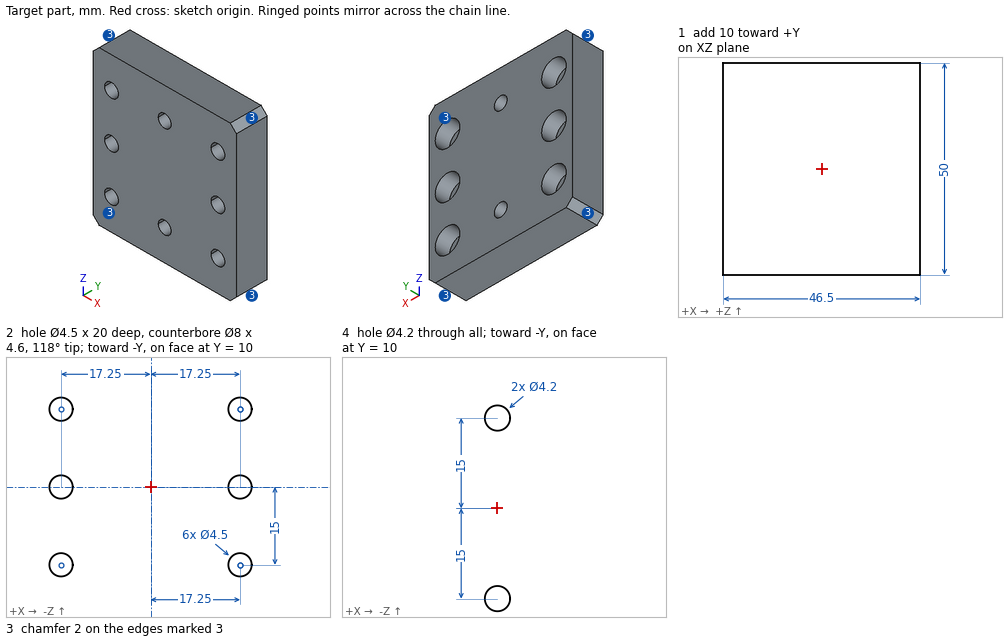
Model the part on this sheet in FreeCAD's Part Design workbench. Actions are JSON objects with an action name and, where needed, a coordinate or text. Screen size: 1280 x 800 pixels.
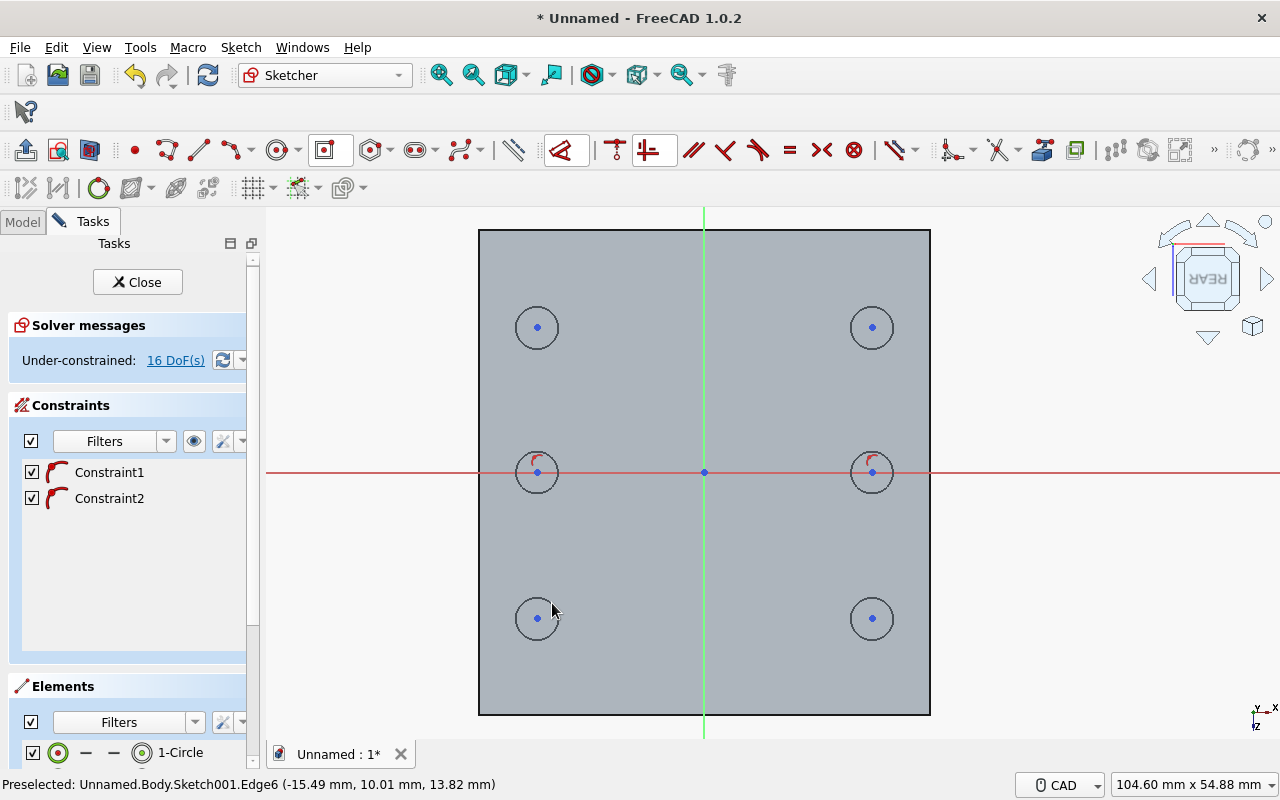
{"action": "left_click", "coordinate": [887, 604]}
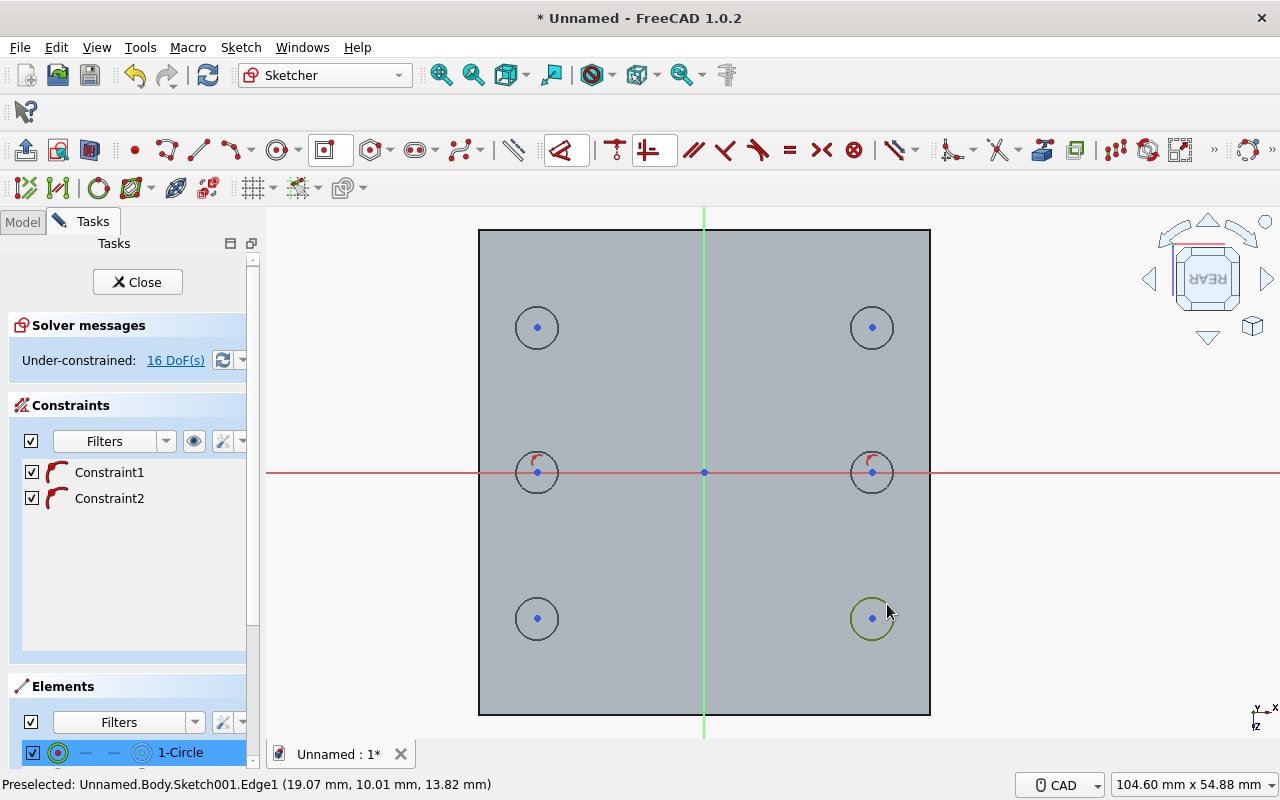
{"action": "left_click", "coordinate": [887, 458]}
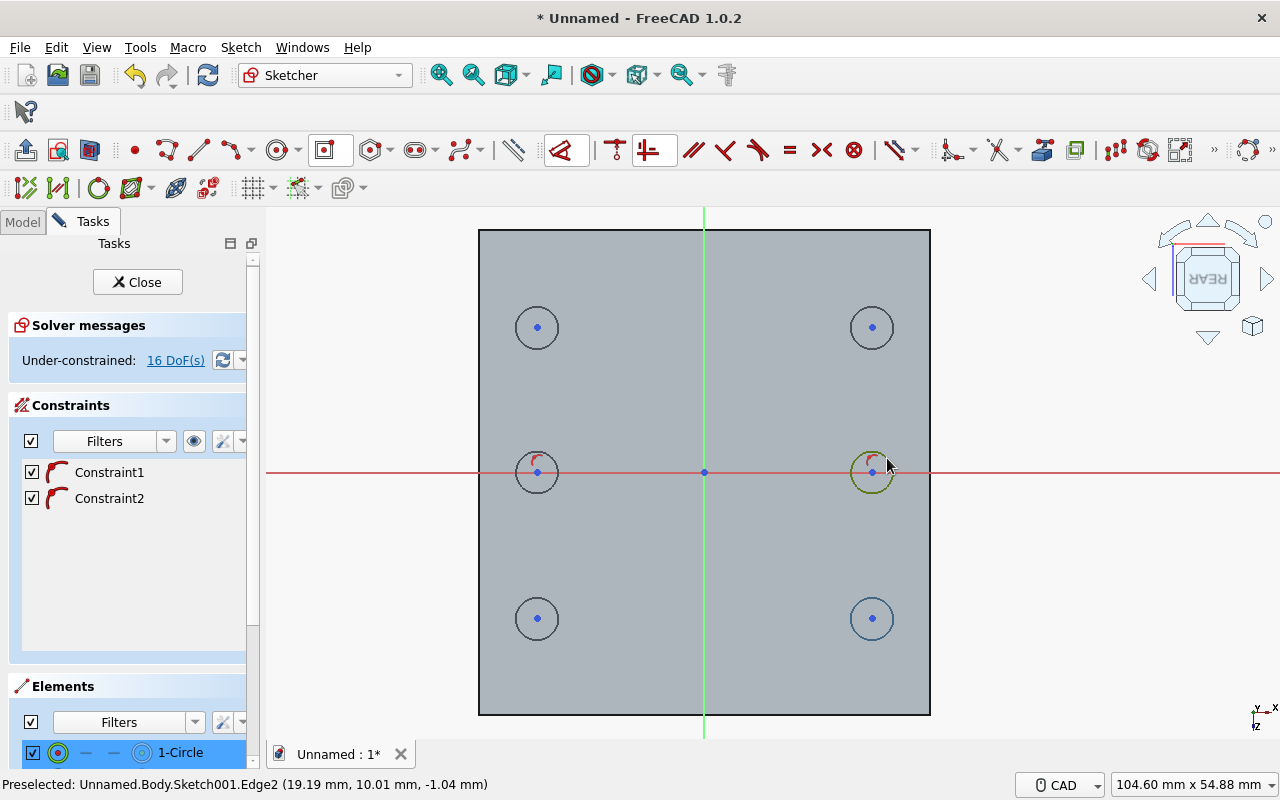
{"action": "left_click", "coordinate": [887, 313]}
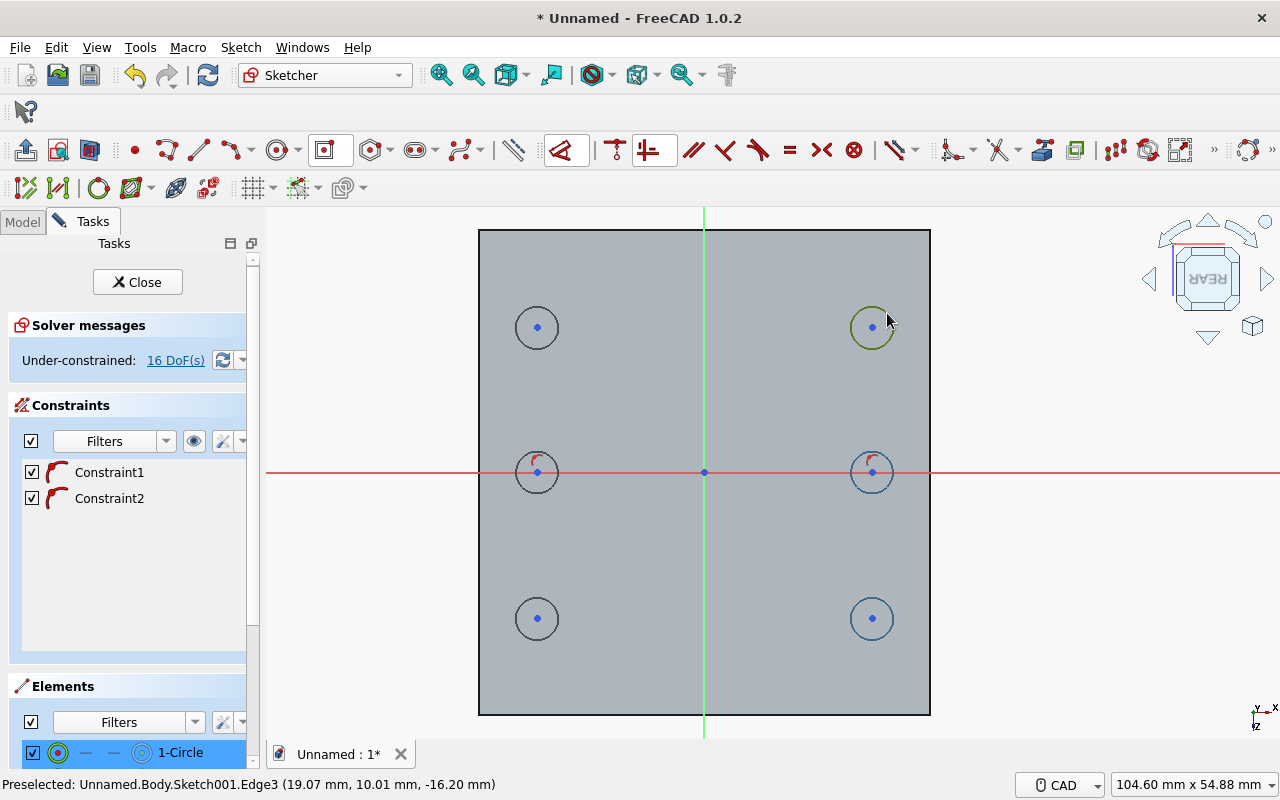
{"action": "left_click", "coordinate": [552, 313]}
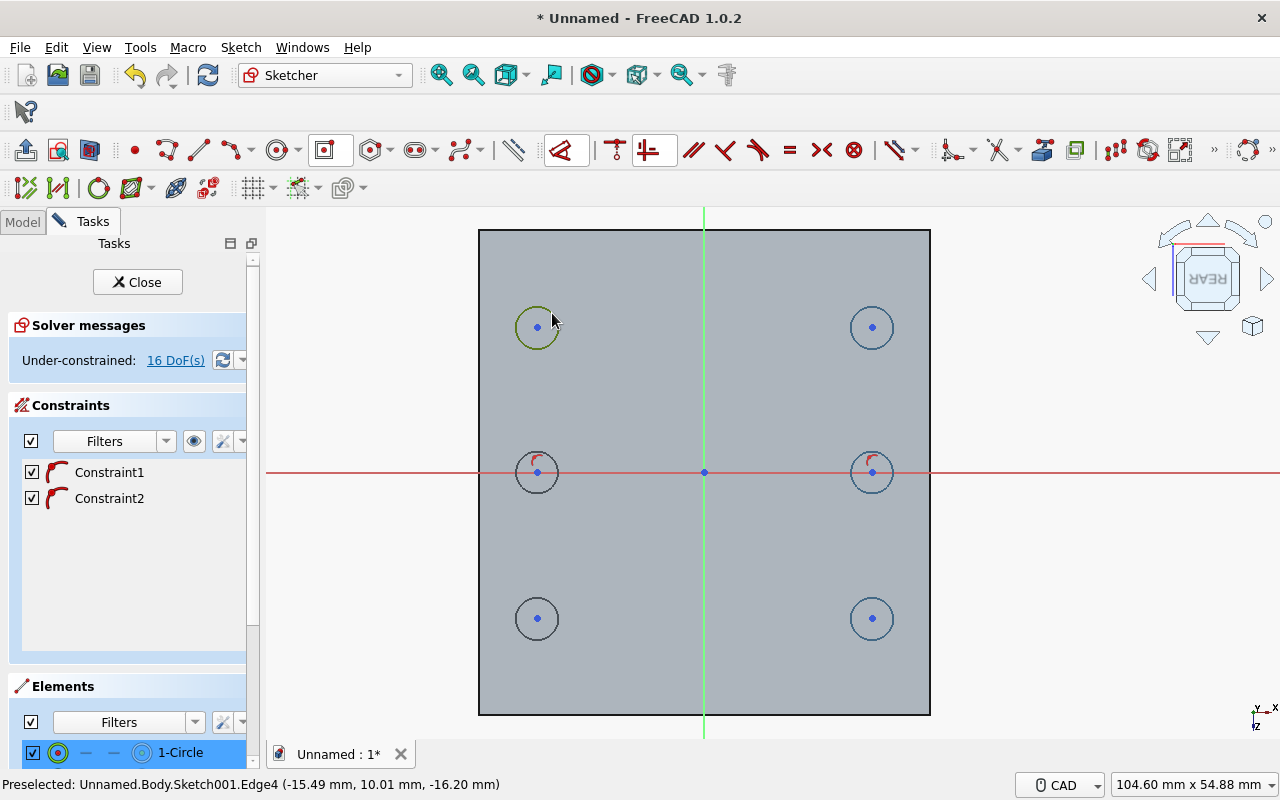
{"action": "left_click", "coordinate": [552, 458]}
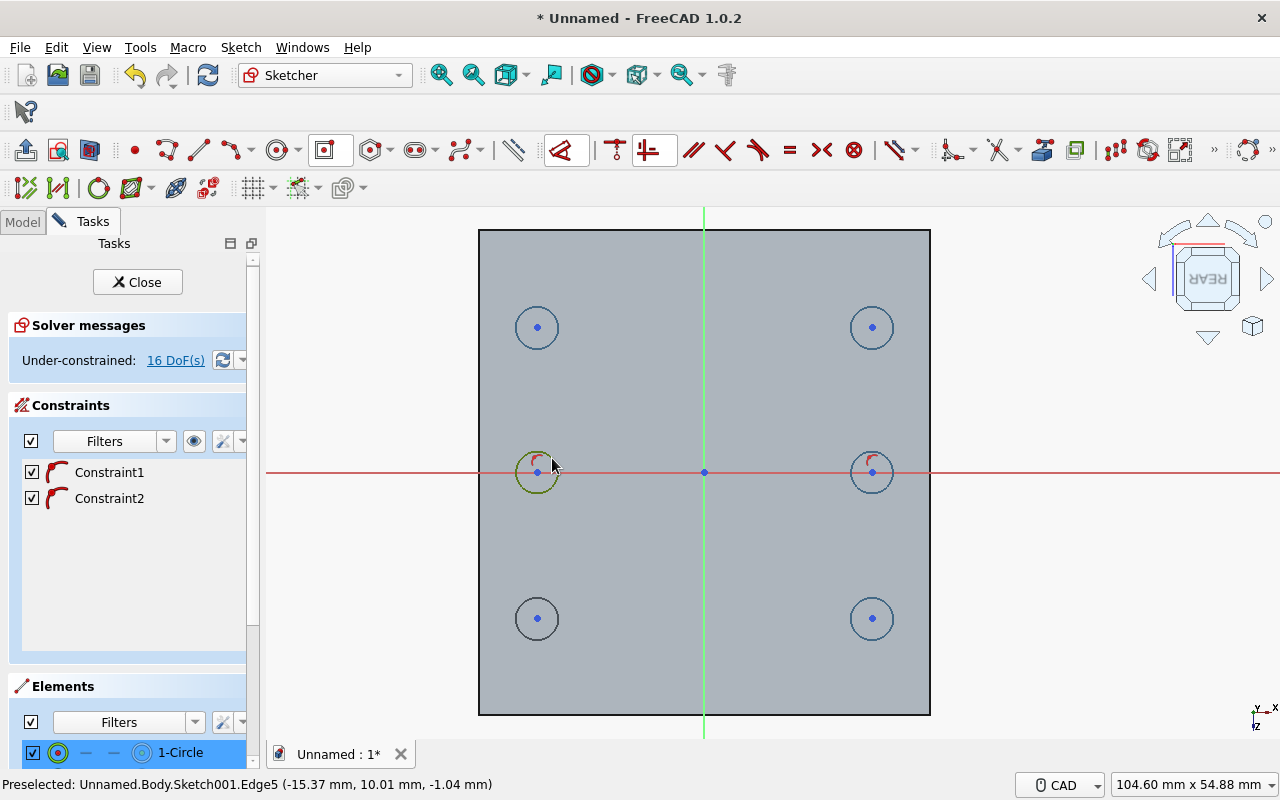
{"action": "left_click", "coordinate": [552, 604]}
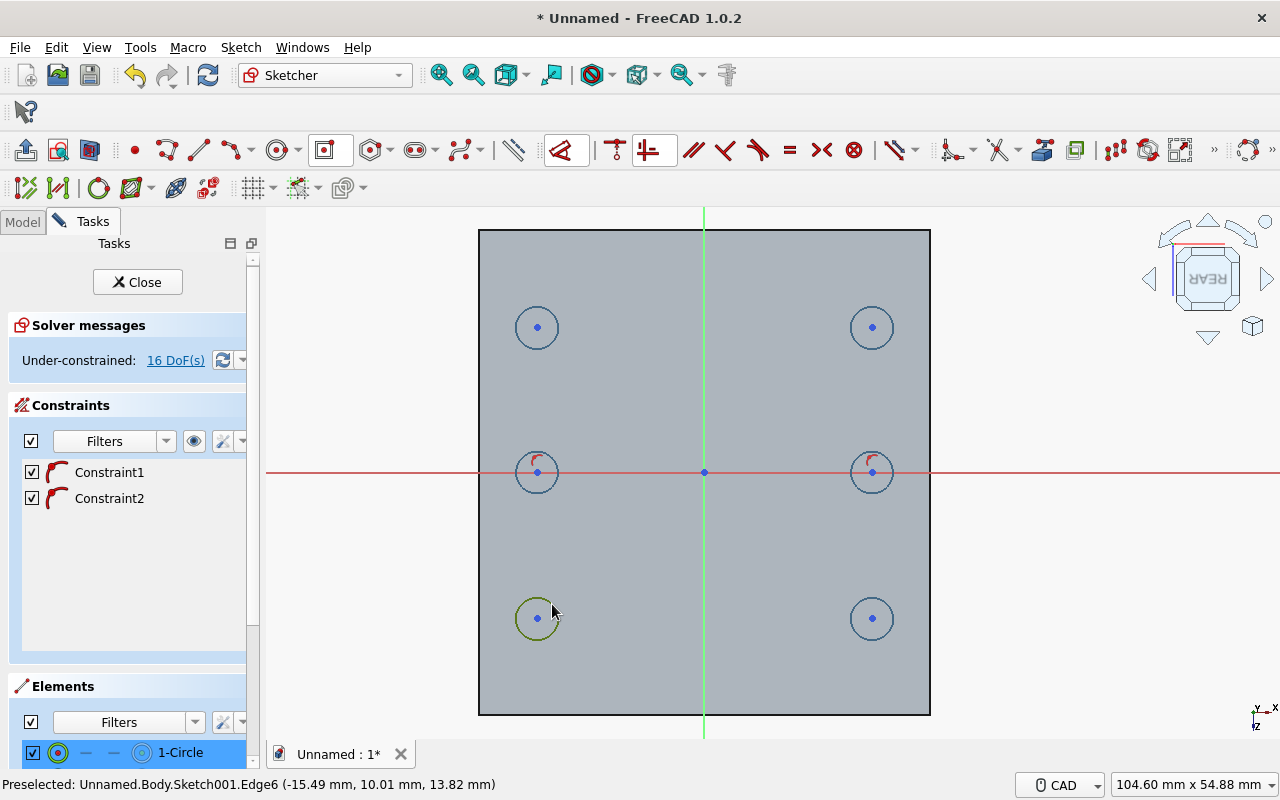
{"action": "left_click", "coordinate": [790, 150]}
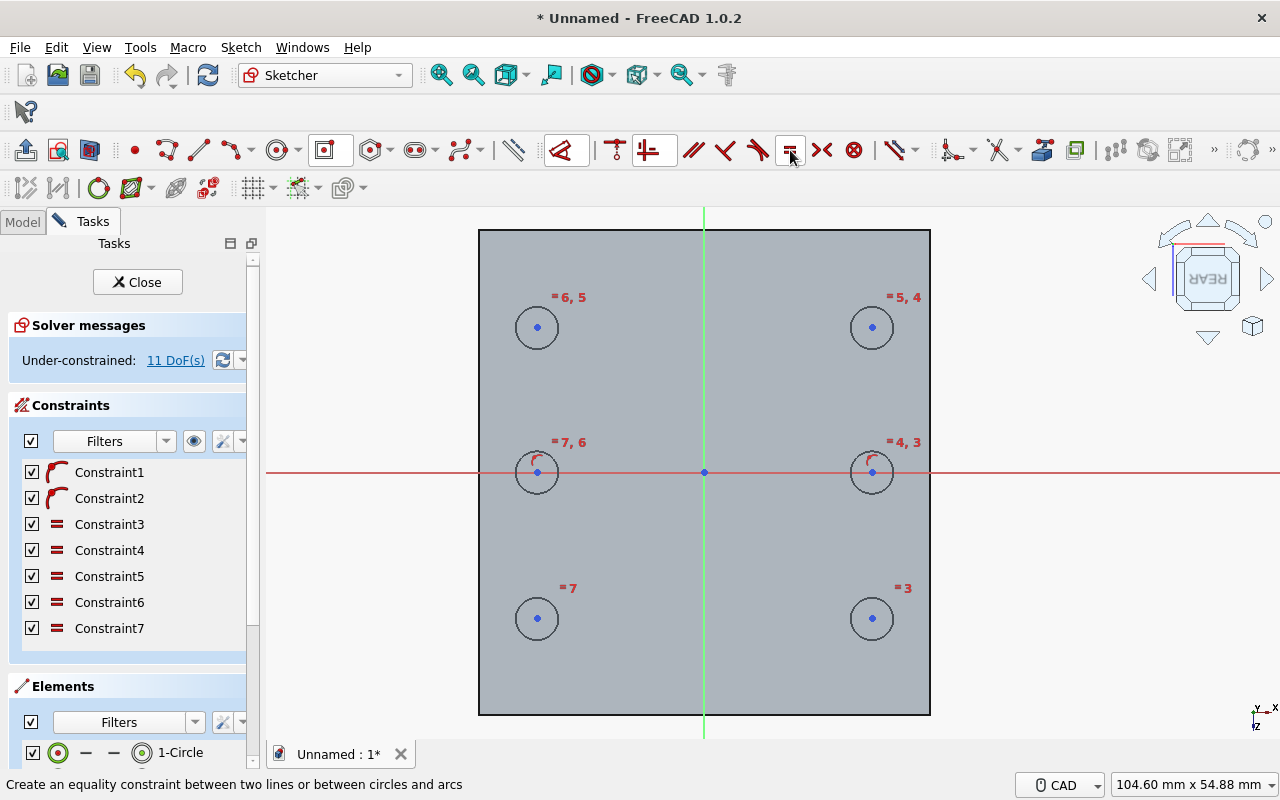
{"action": "left_click", "coordinate": [872, 619]}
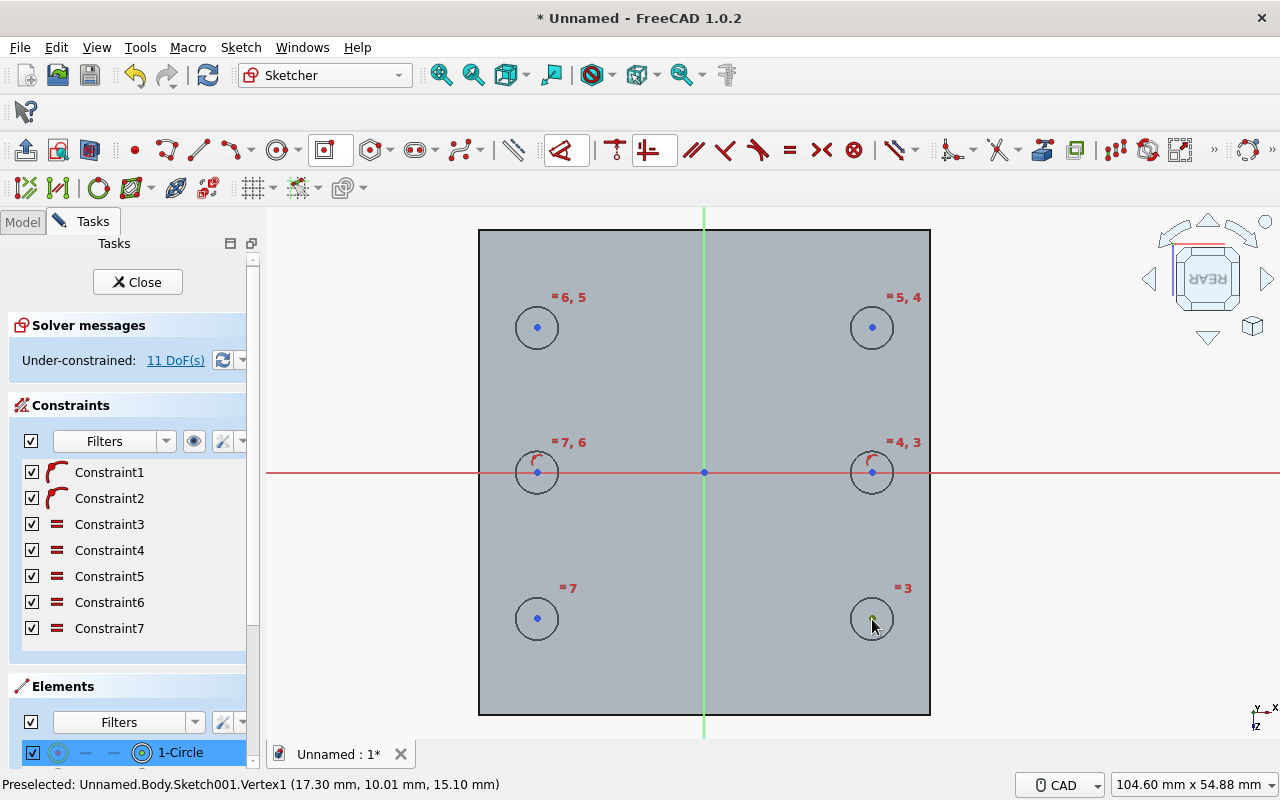
{"action": "left_click", "coordinate": [872, 328]}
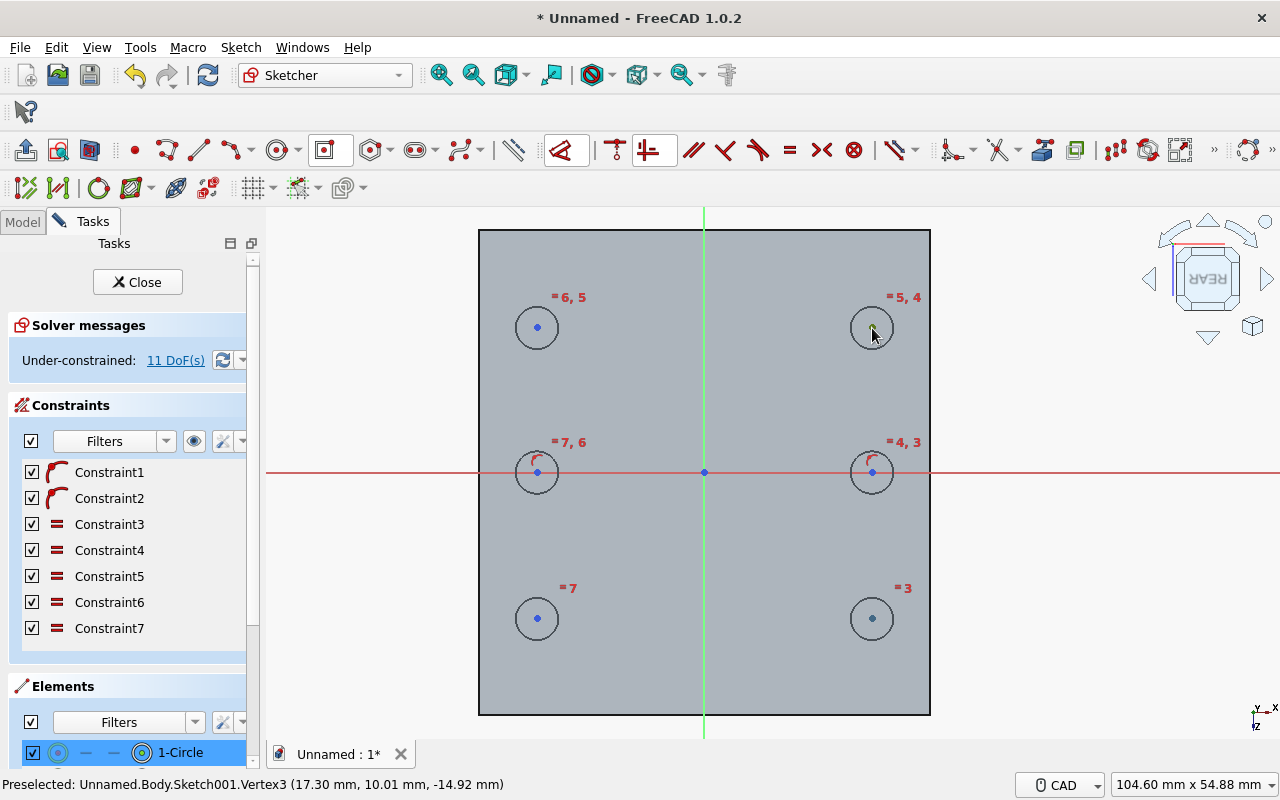
{"action": "left_click", "coordinate": [353, 473]}